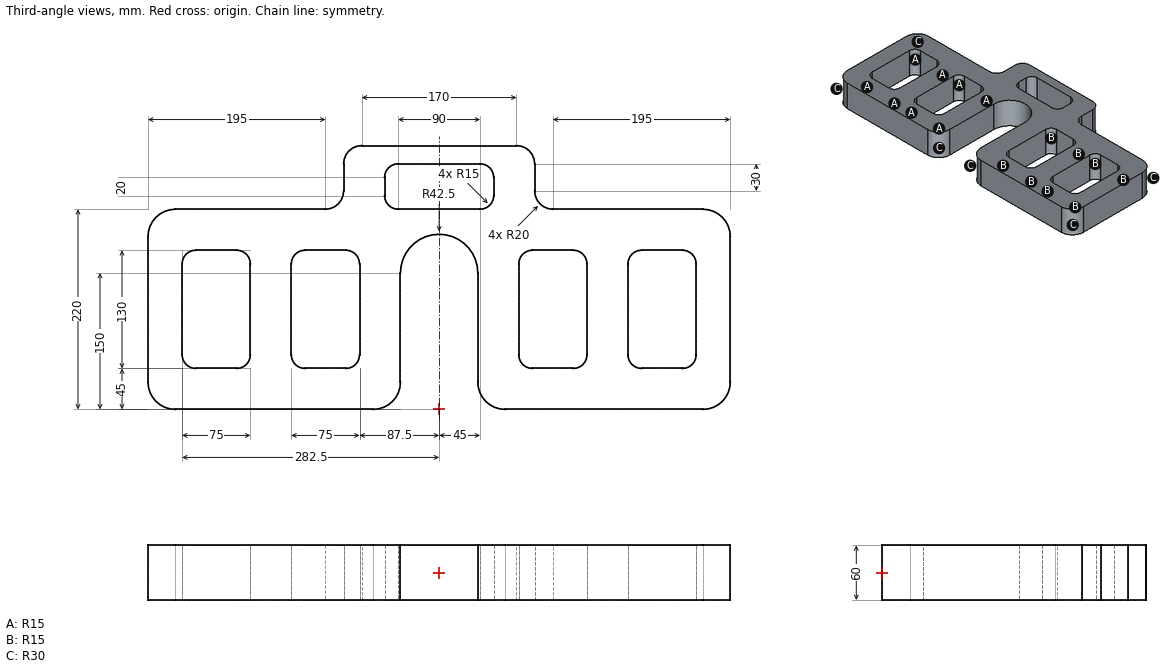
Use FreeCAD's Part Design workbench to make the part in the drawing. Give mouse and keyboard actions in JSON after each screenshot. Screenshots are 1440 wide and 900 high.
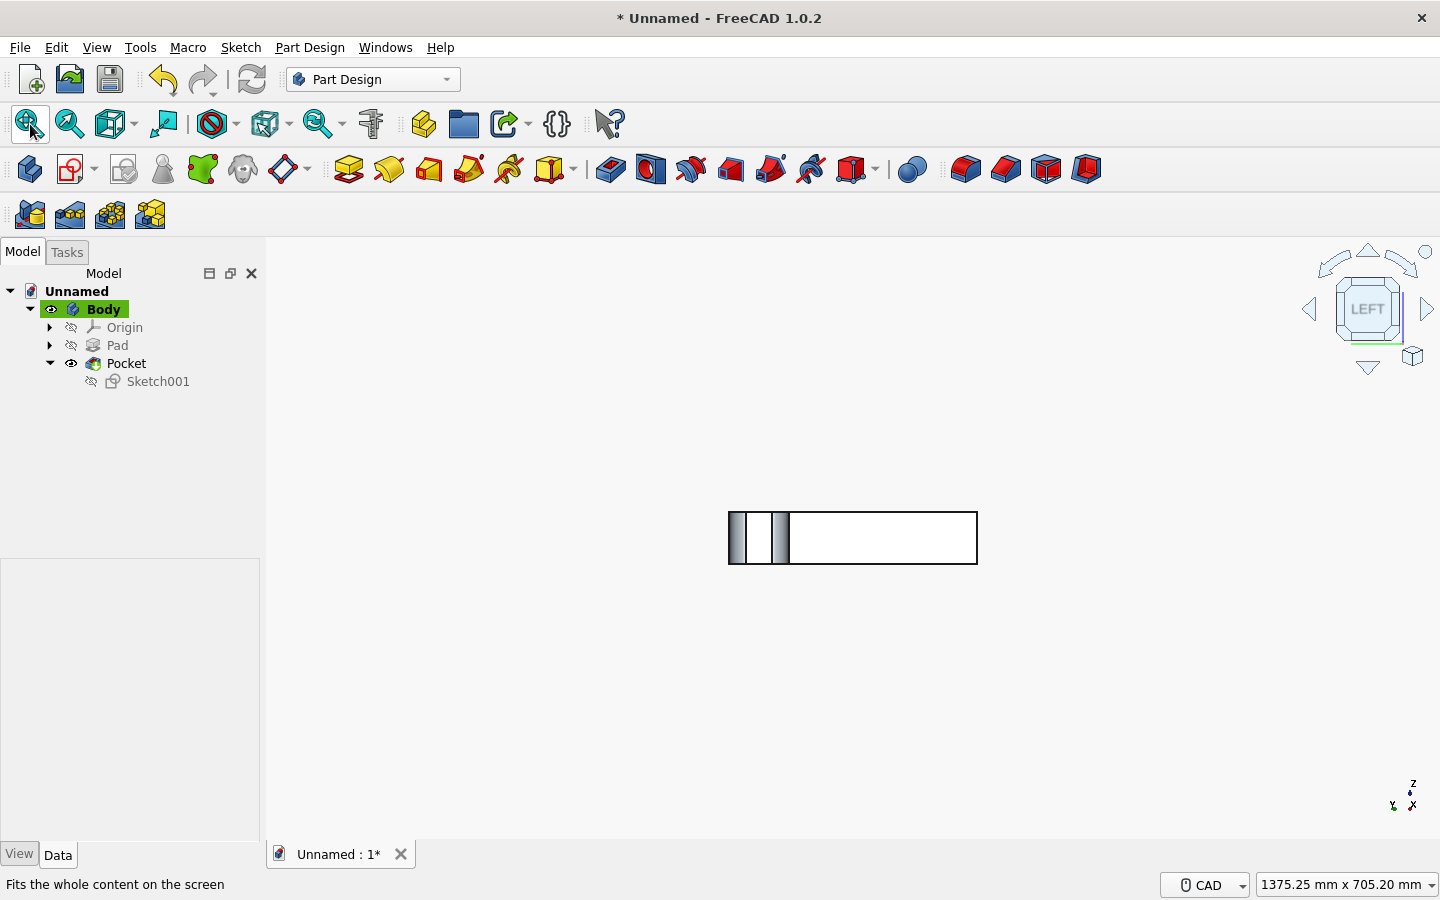
{"action": "key", "text": "v 3"}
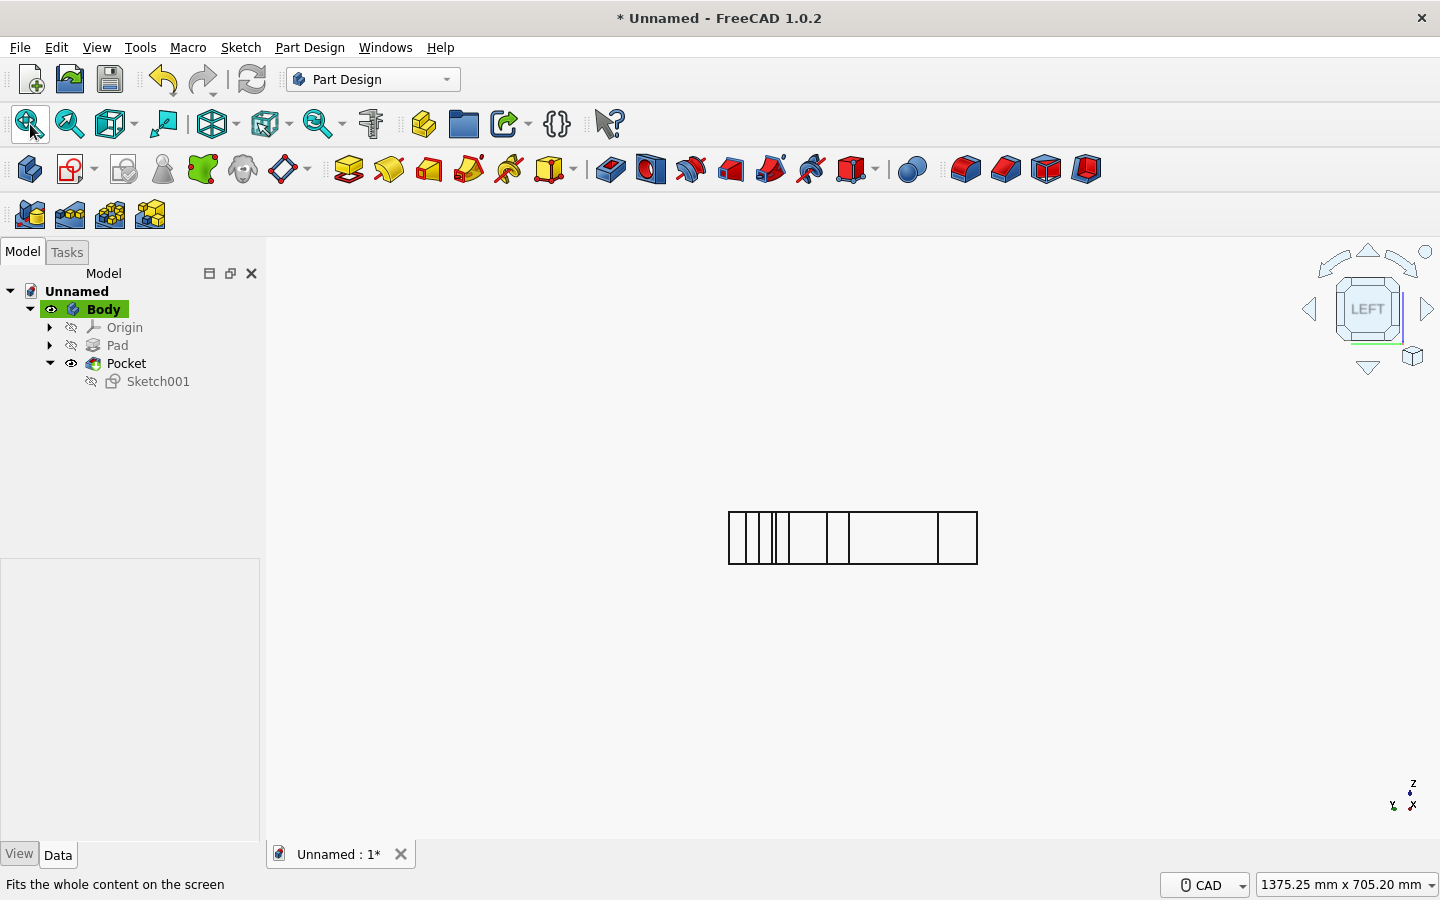
{"action": "key", "text": "0"}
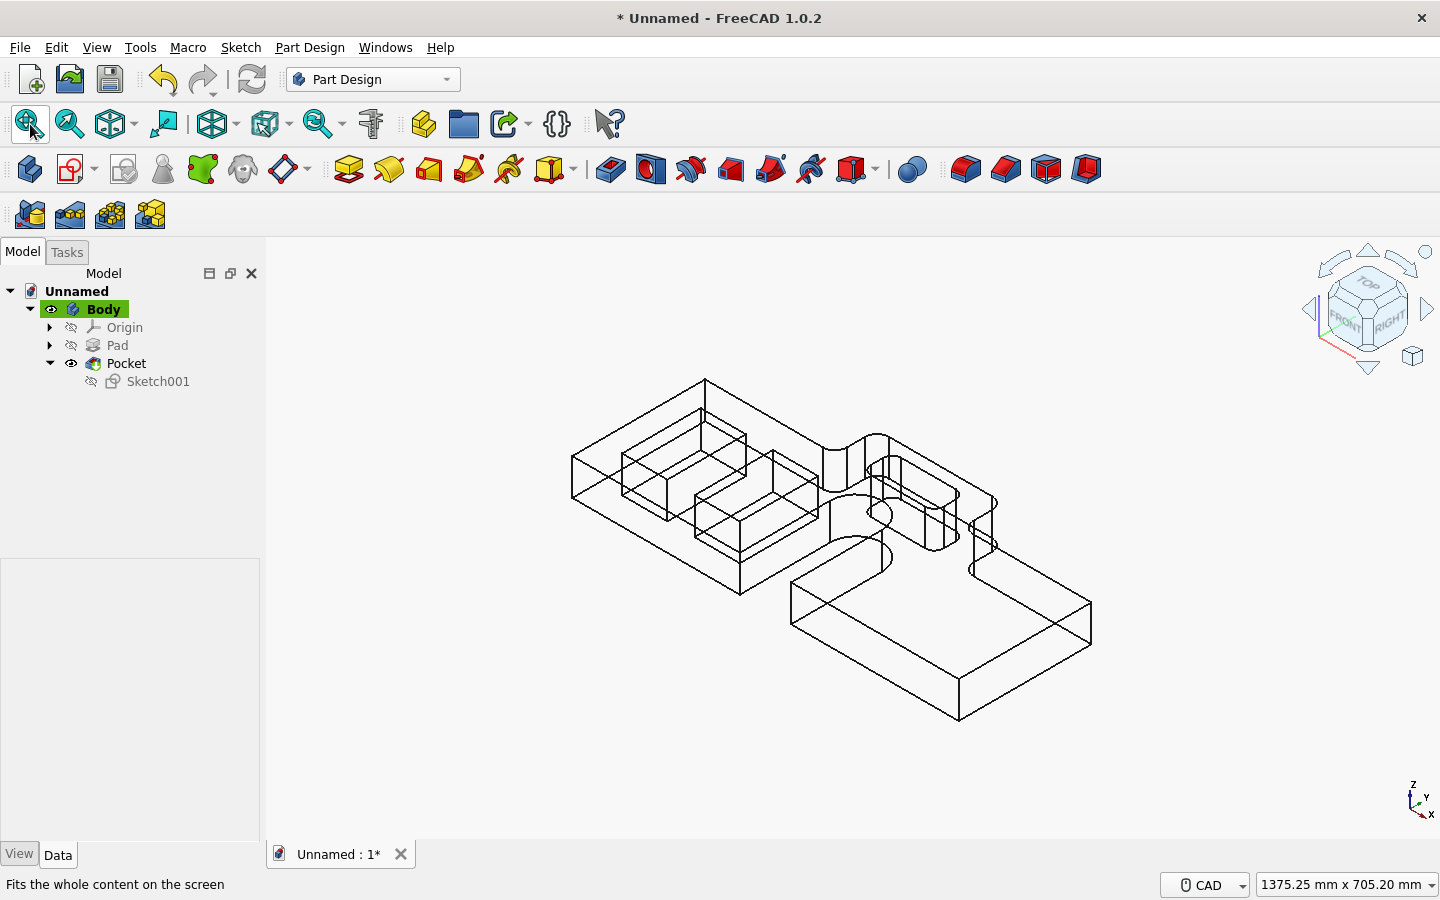
{"action": "left_click", "coordinate": [746, 454]}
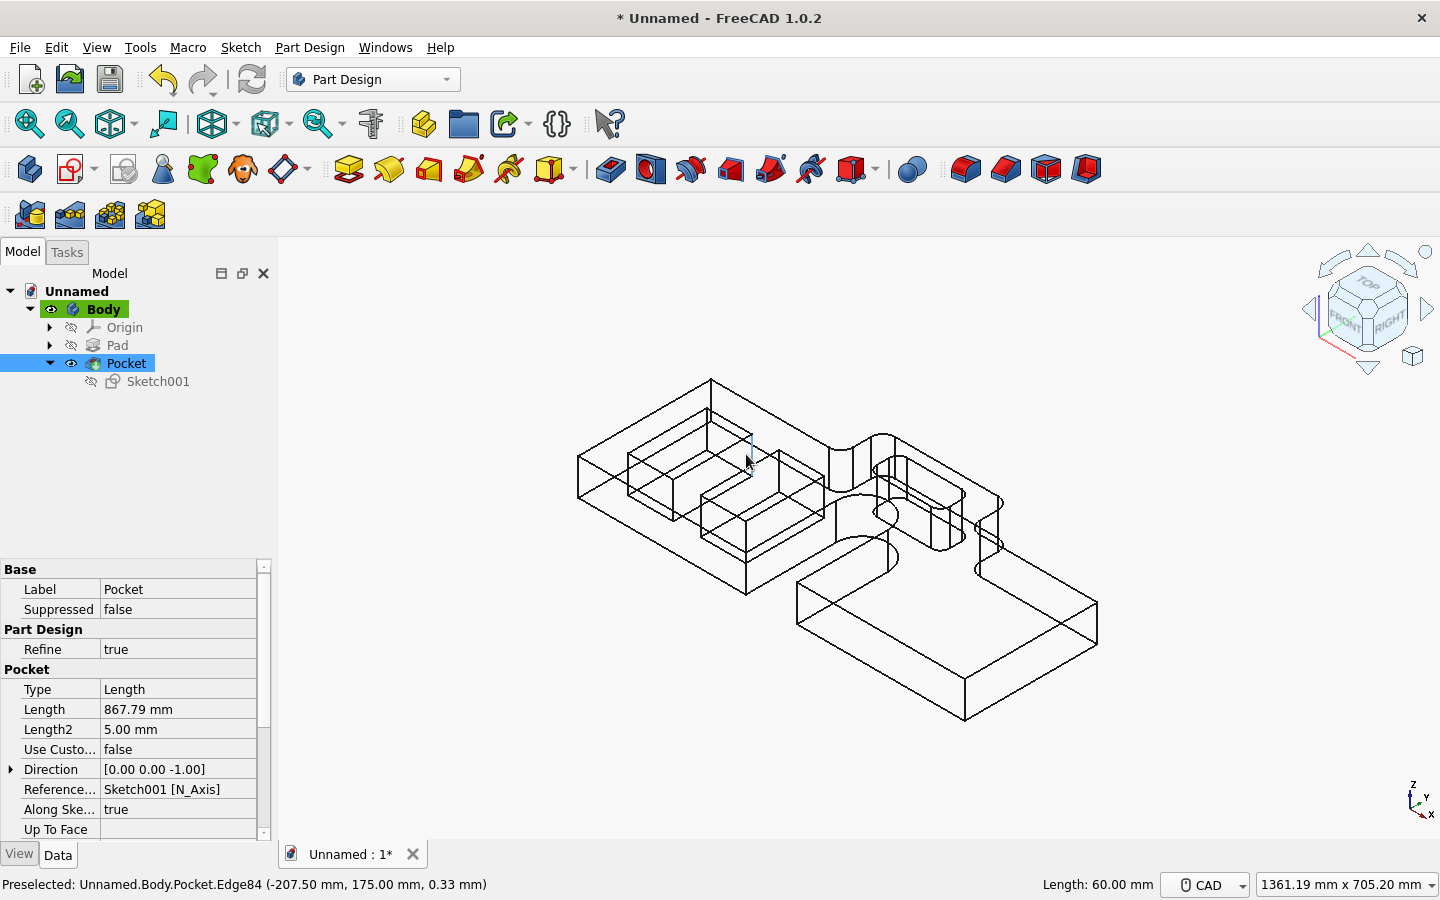
{"action": "left_click", "coordinate": [673, 500], "text": "ctrl"}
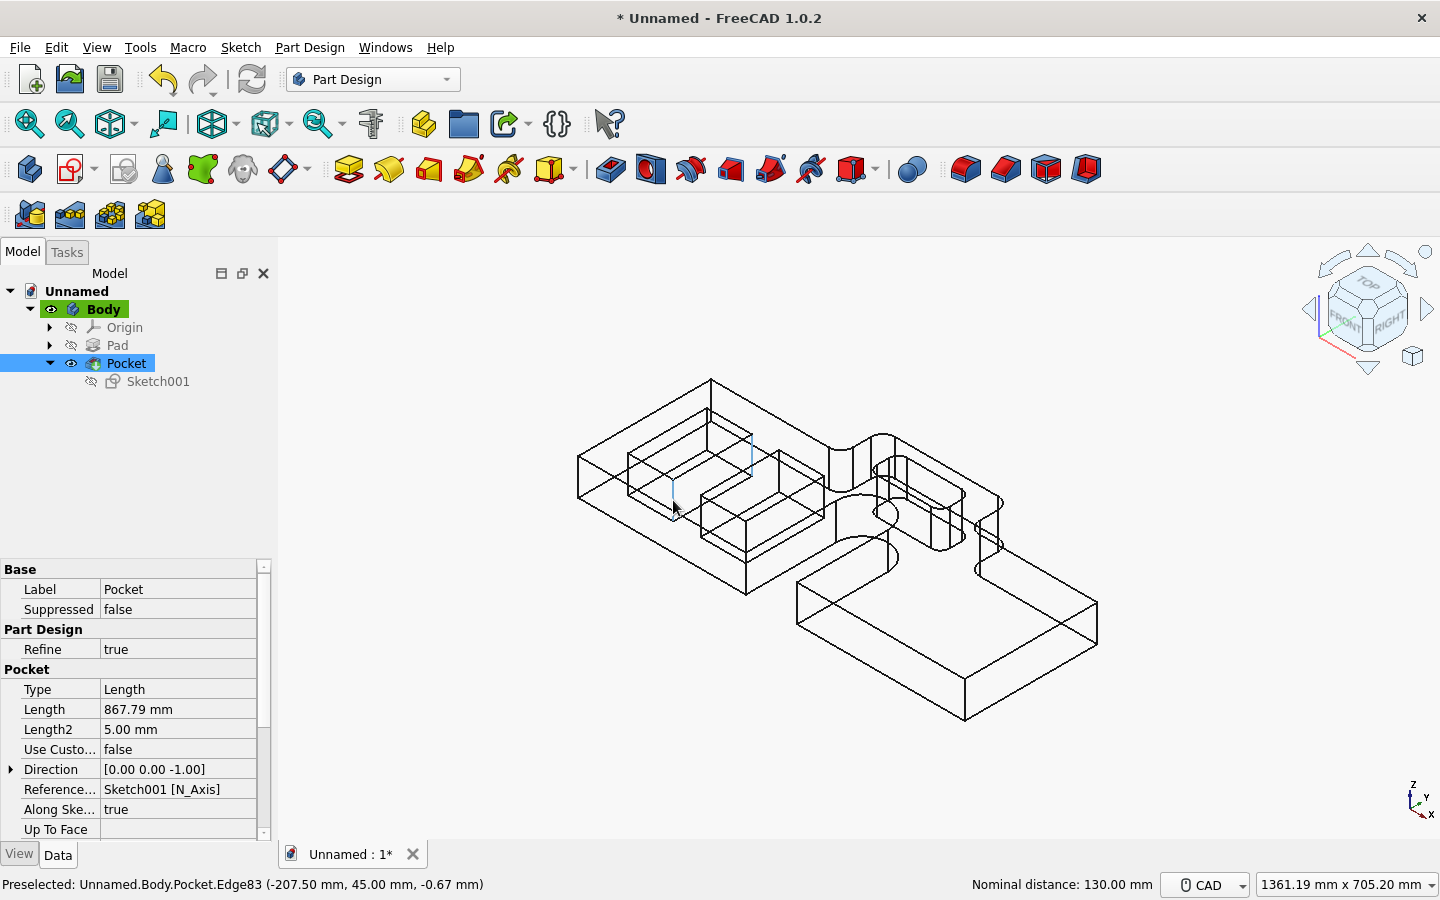
{"action": "left_click", "coordinate": [628, 473], "text": "ctrl"}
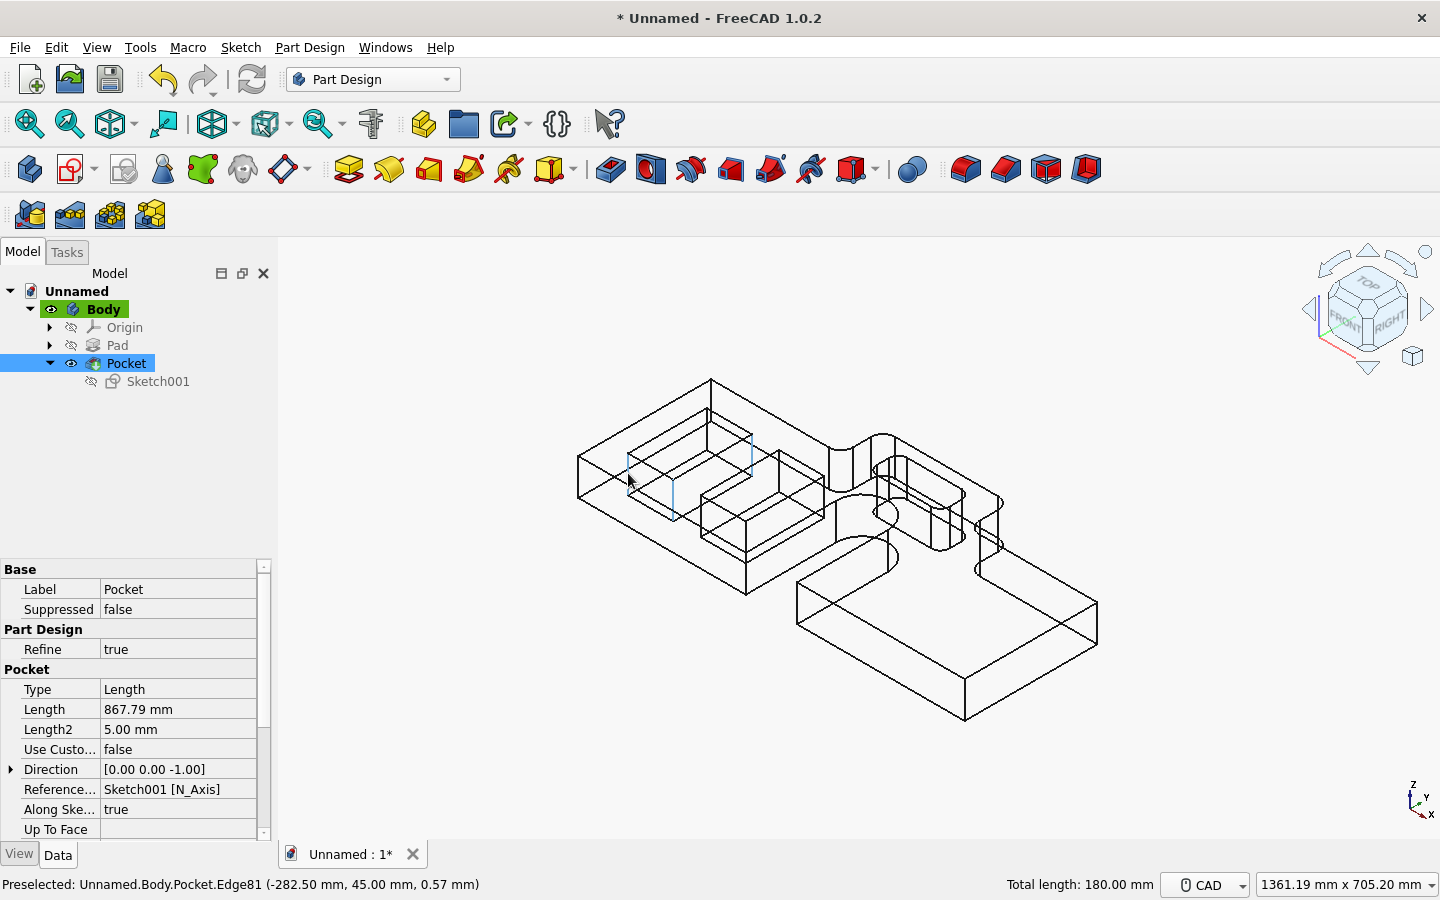
{"action": "left_click", "coordinate": [707, 428], "text": "ctrl"}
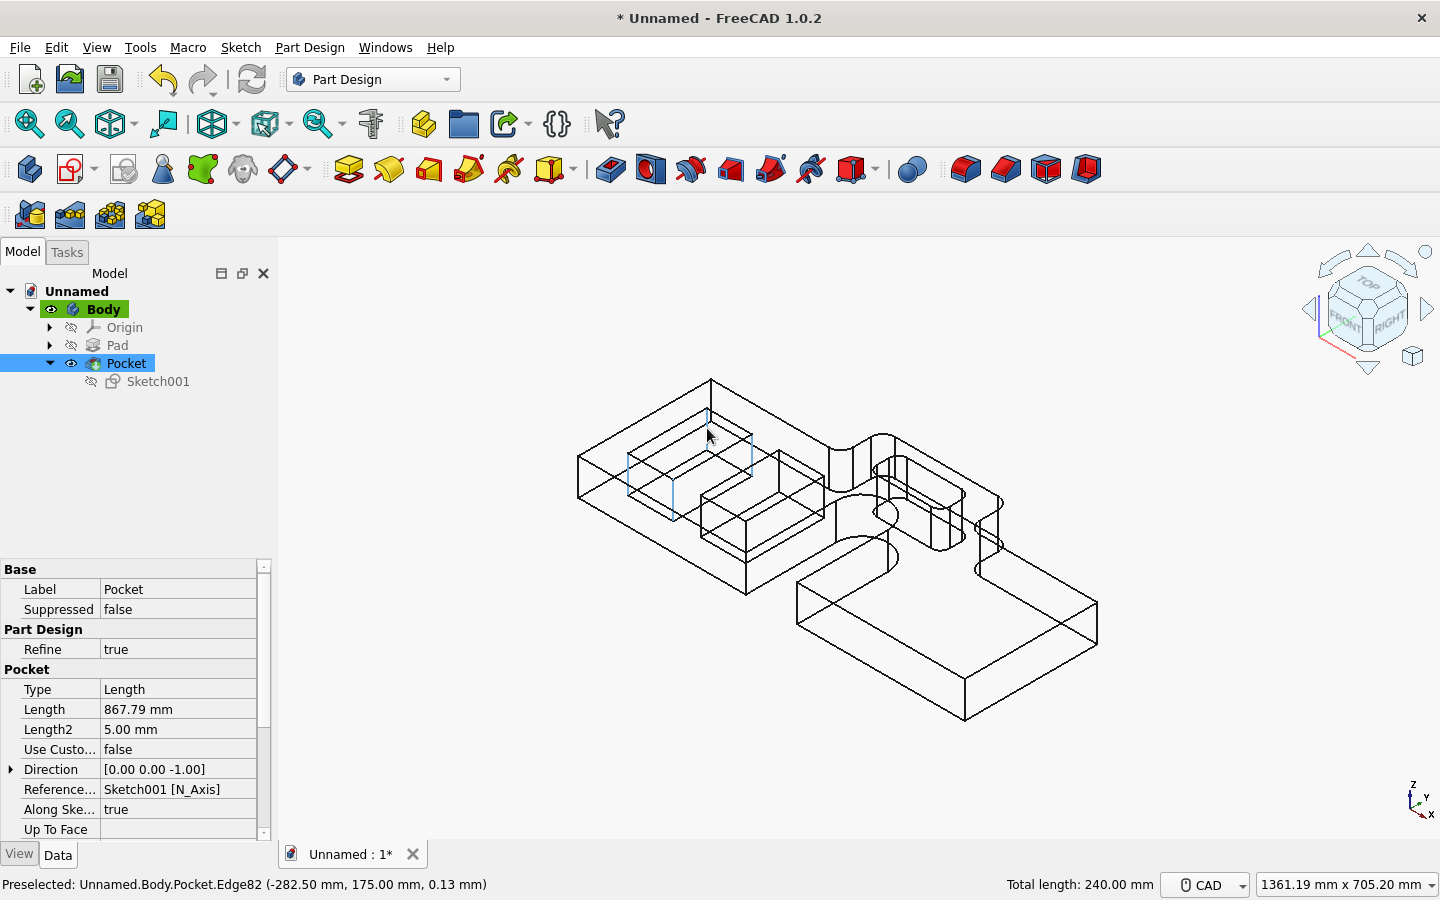
{"action": "left_click", "coordinate": [824, 496], "text": "ctrl"}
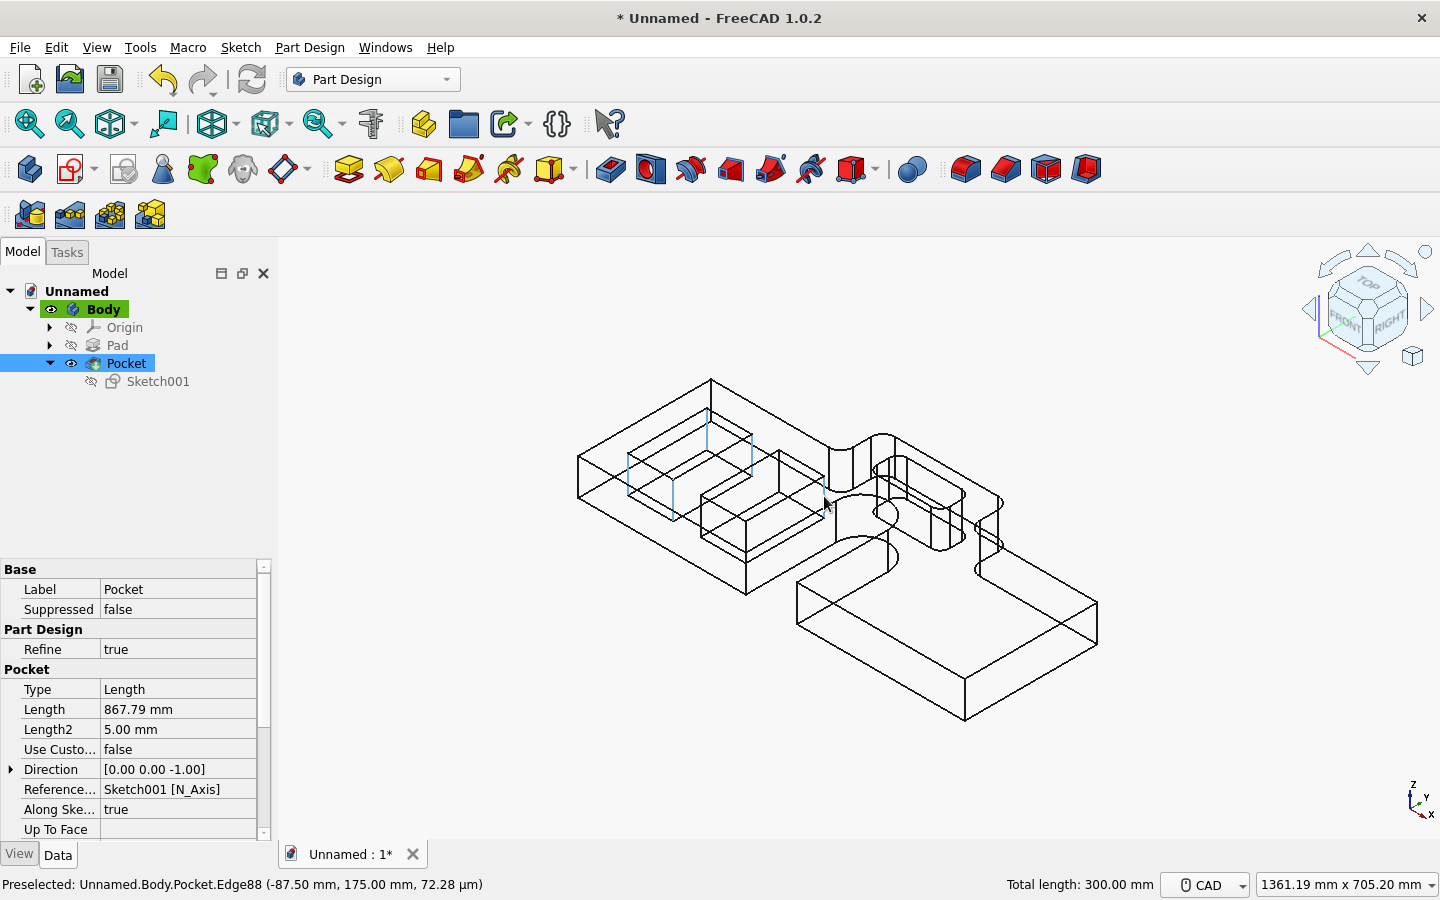
{"action": "left_click", "coordinate": [746, 541], "text": "ctrl"}